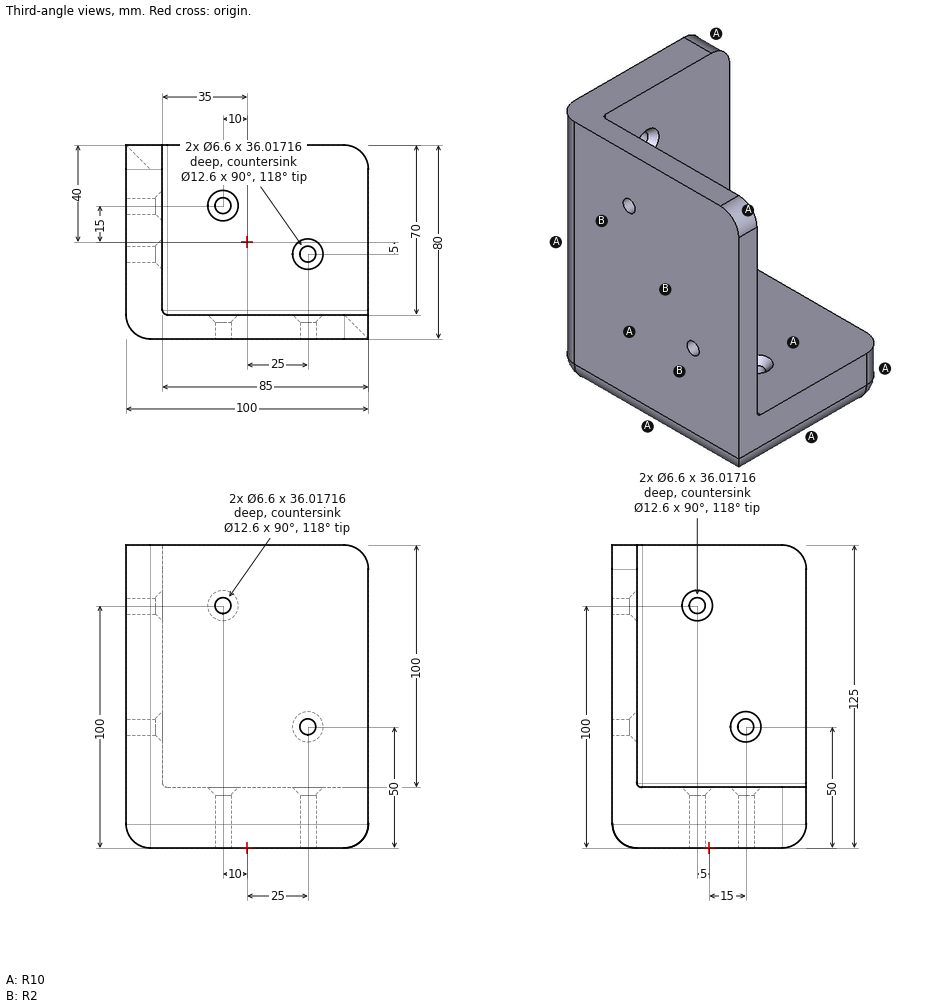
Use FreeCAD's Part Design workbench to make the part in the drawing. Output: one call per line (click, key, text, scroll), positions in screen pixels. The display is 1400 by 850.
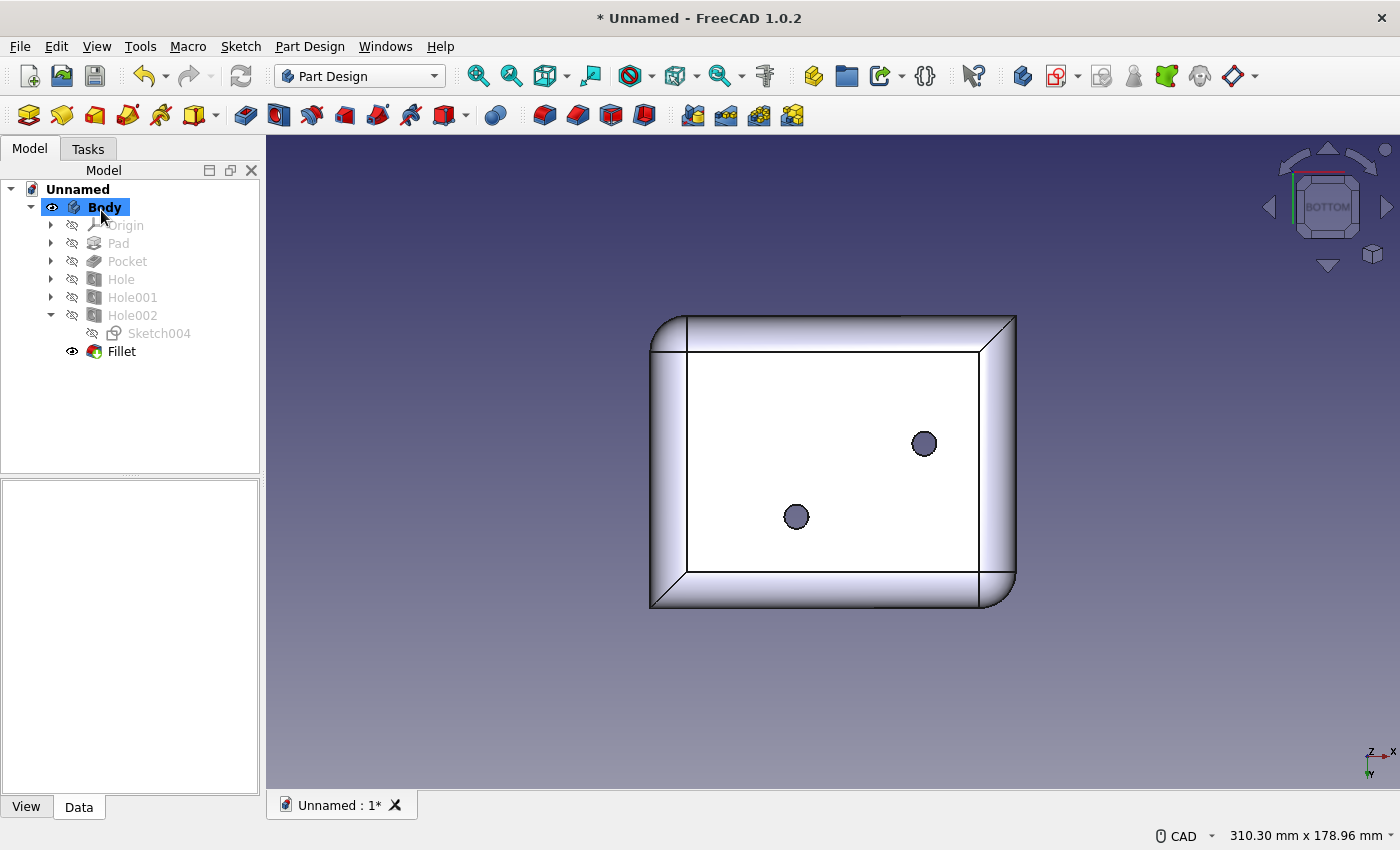
key(0)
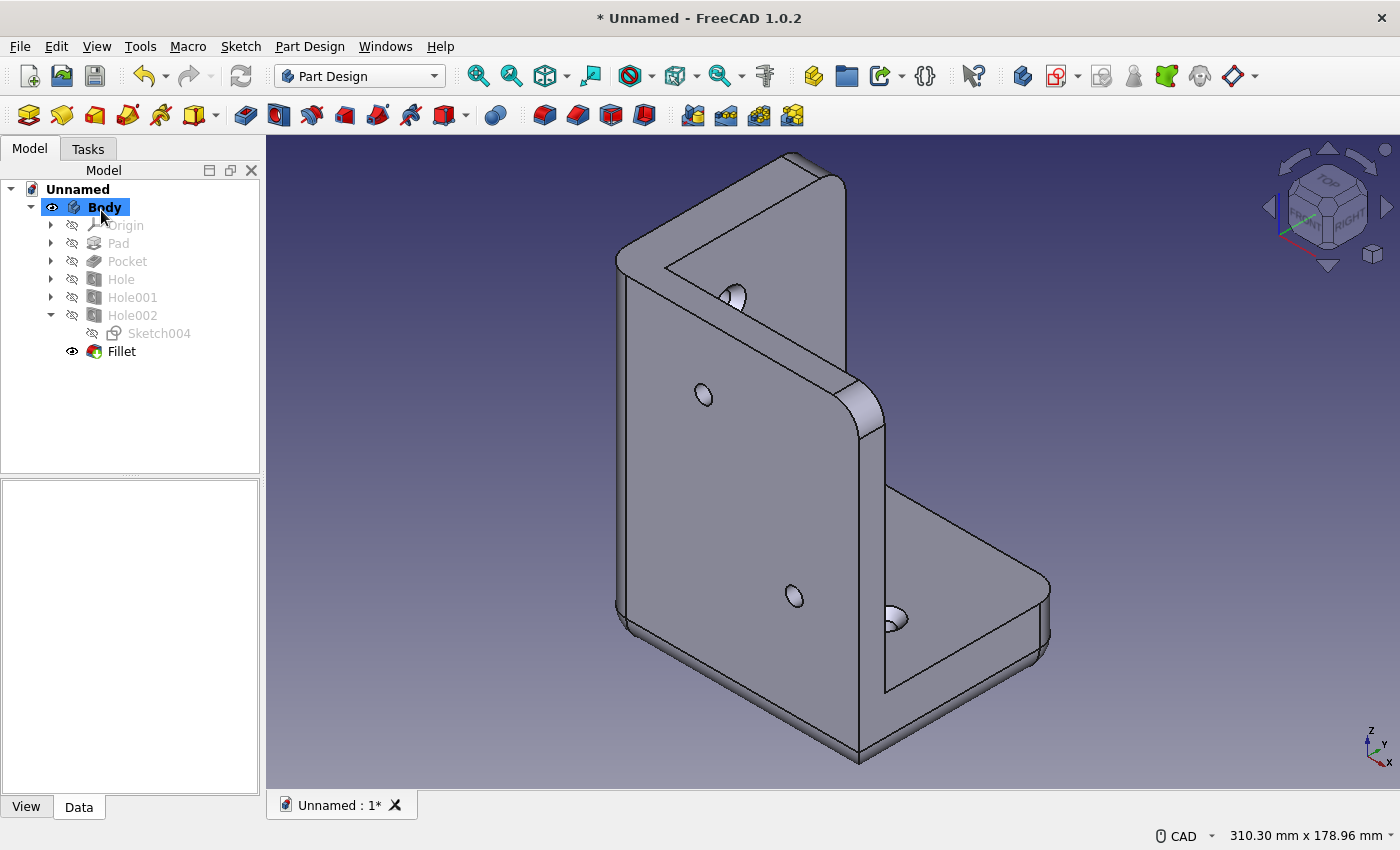
key(2)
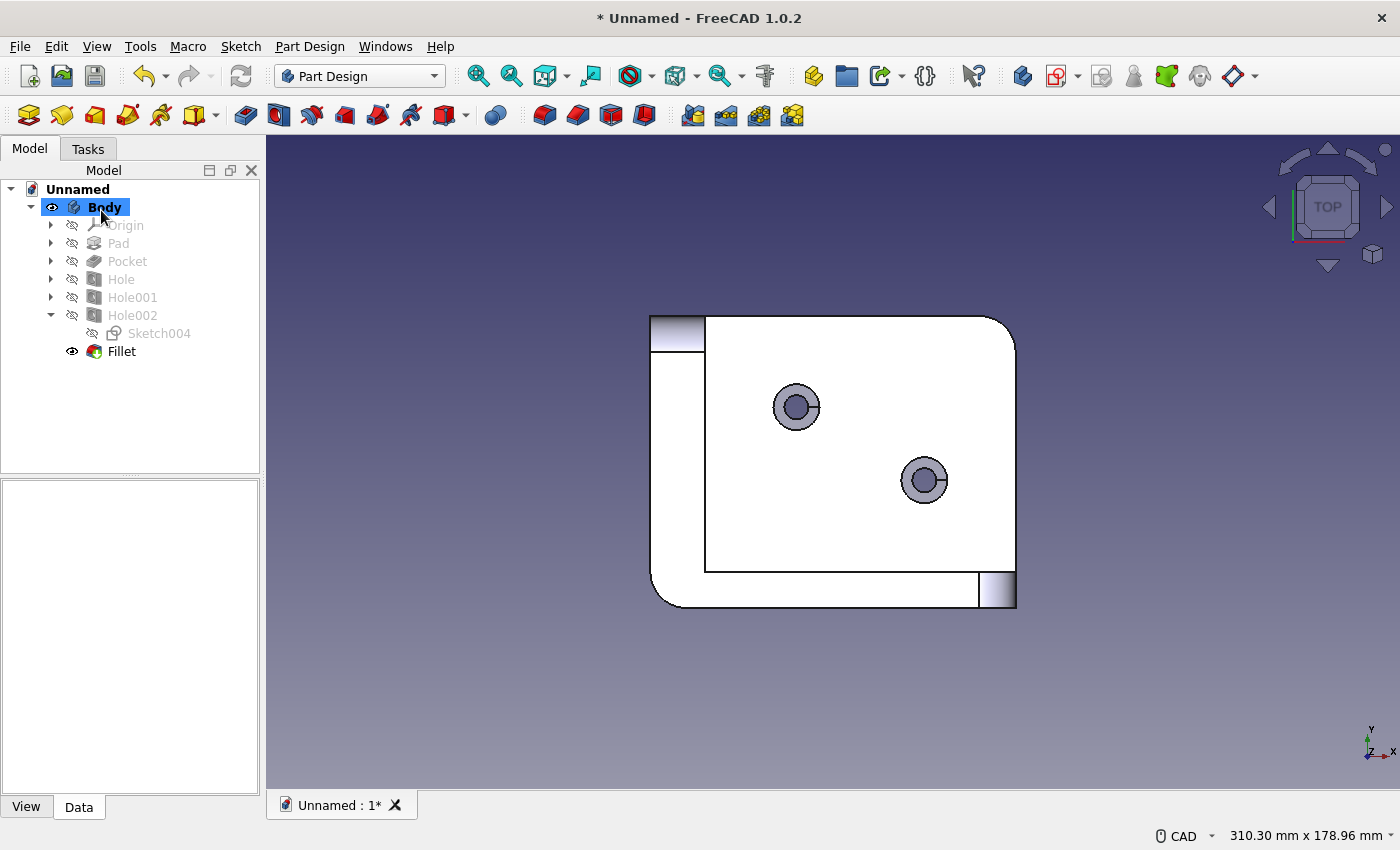
click(479, 76)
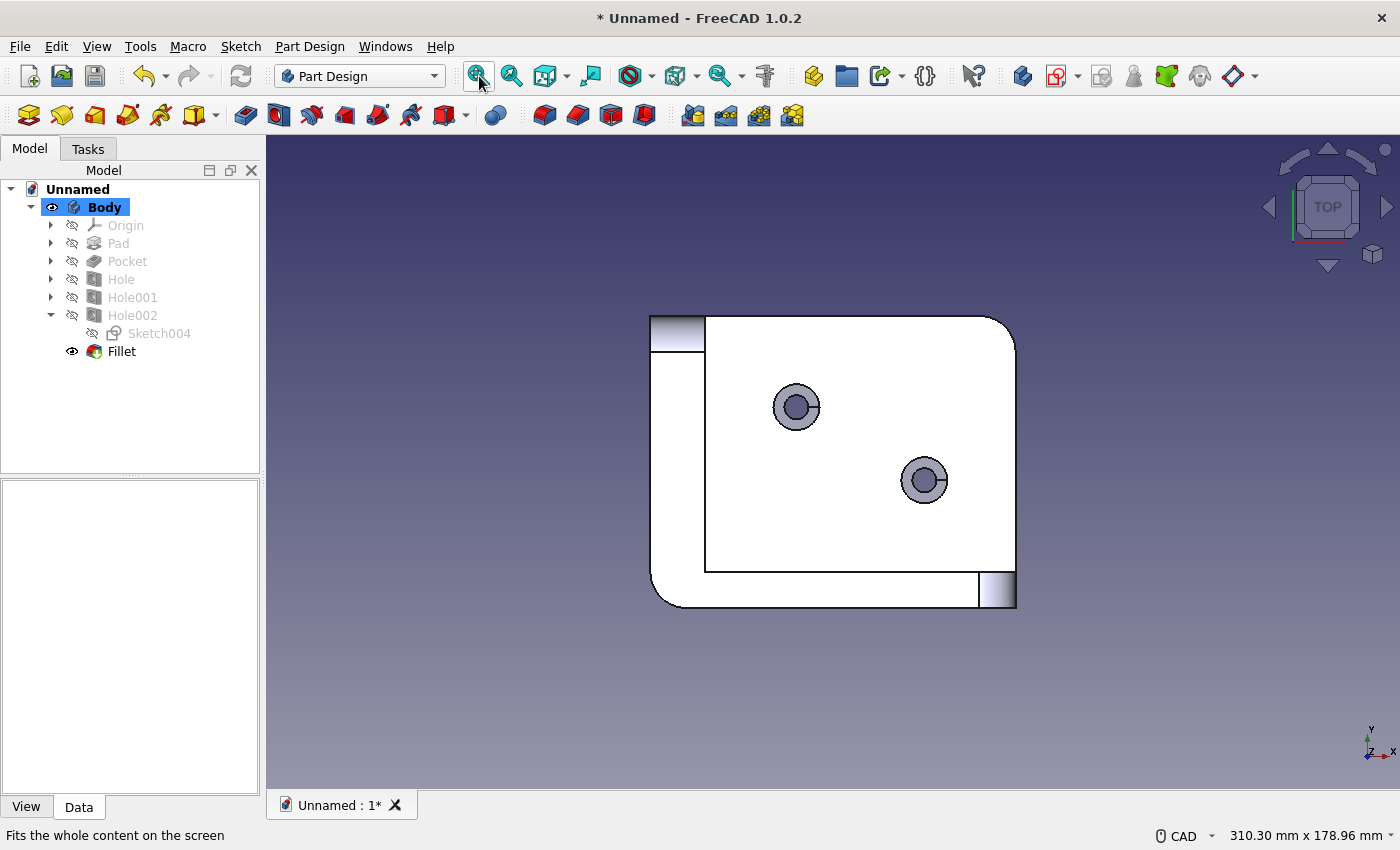
key(1)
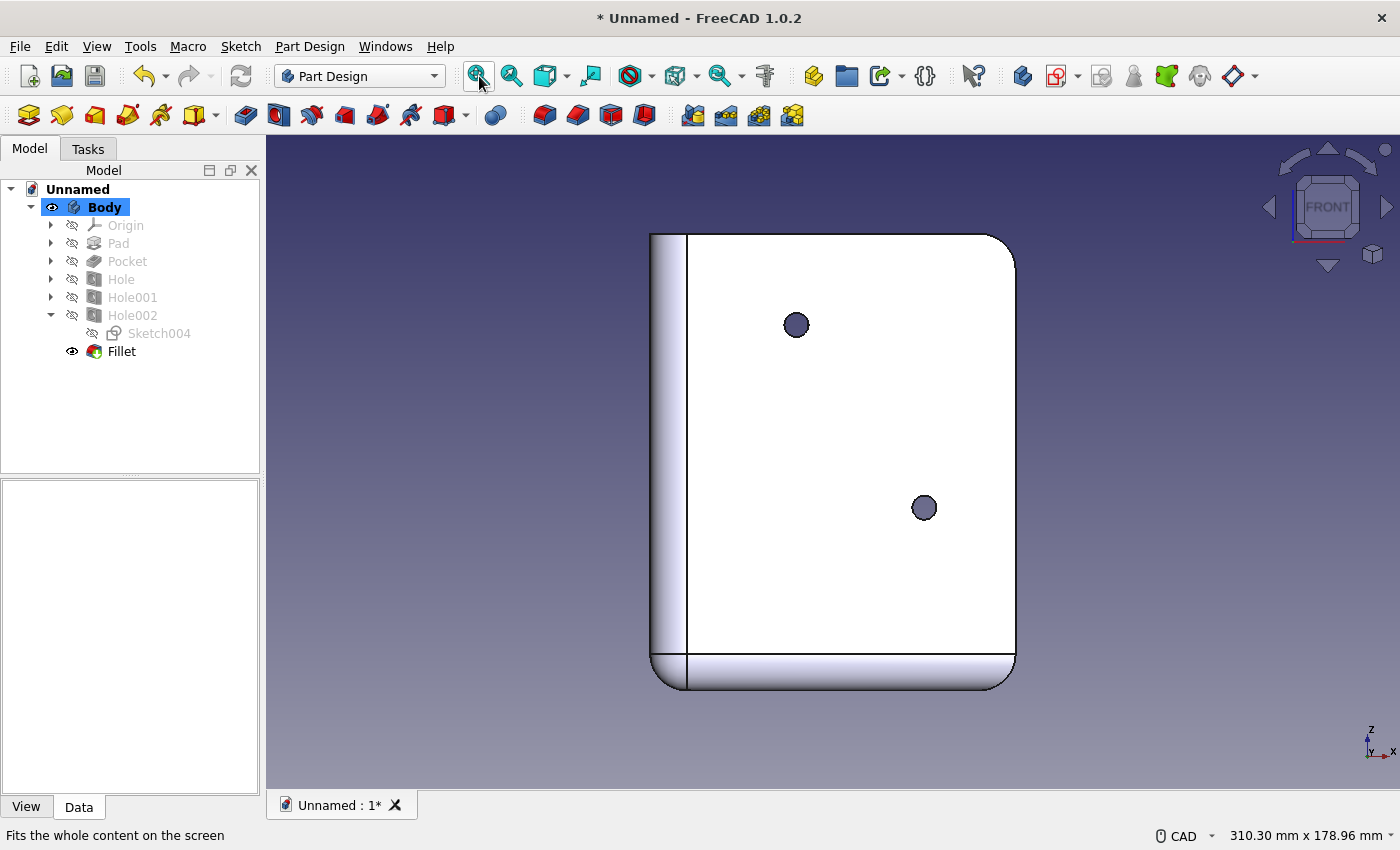
key(3)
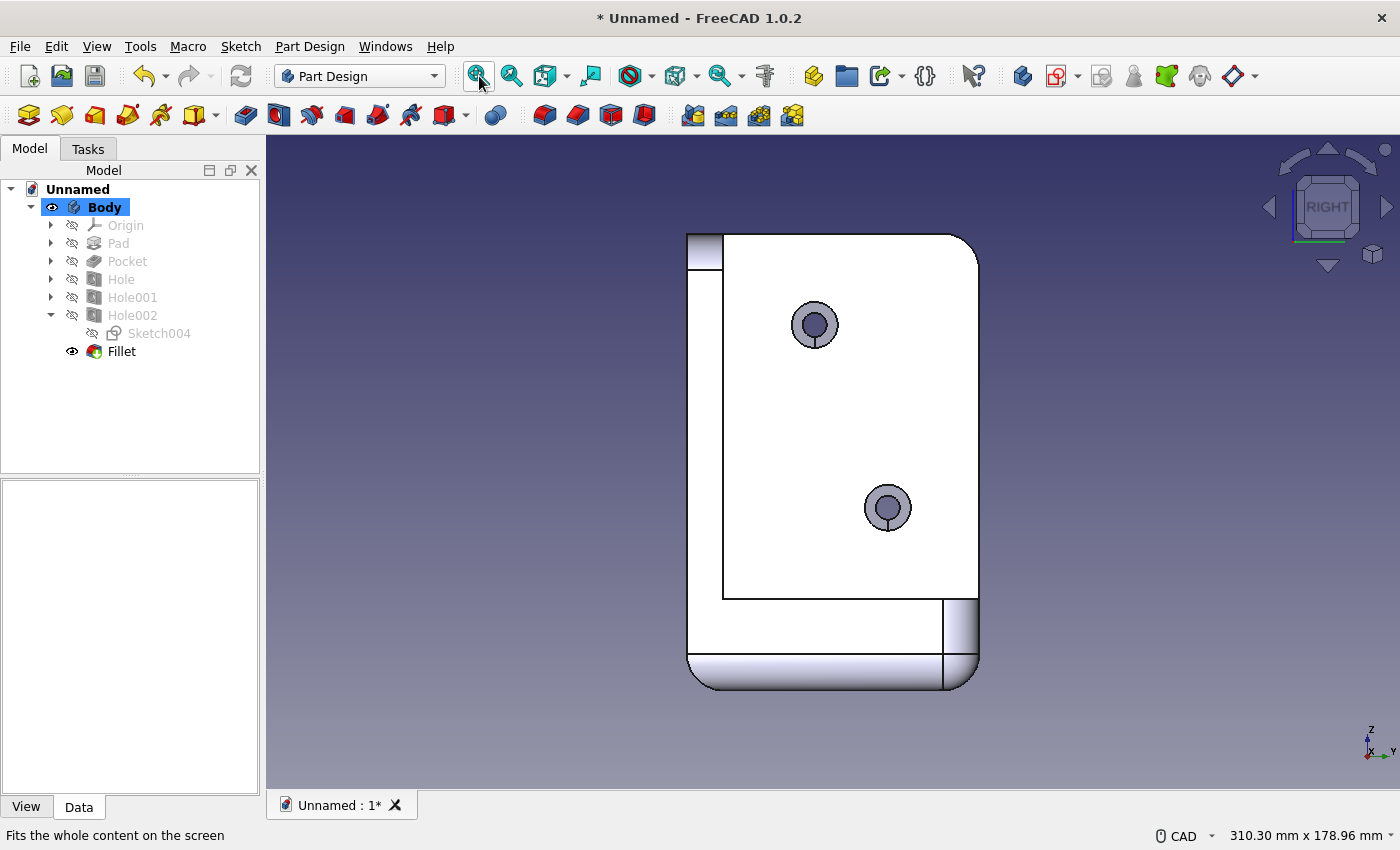
key(5)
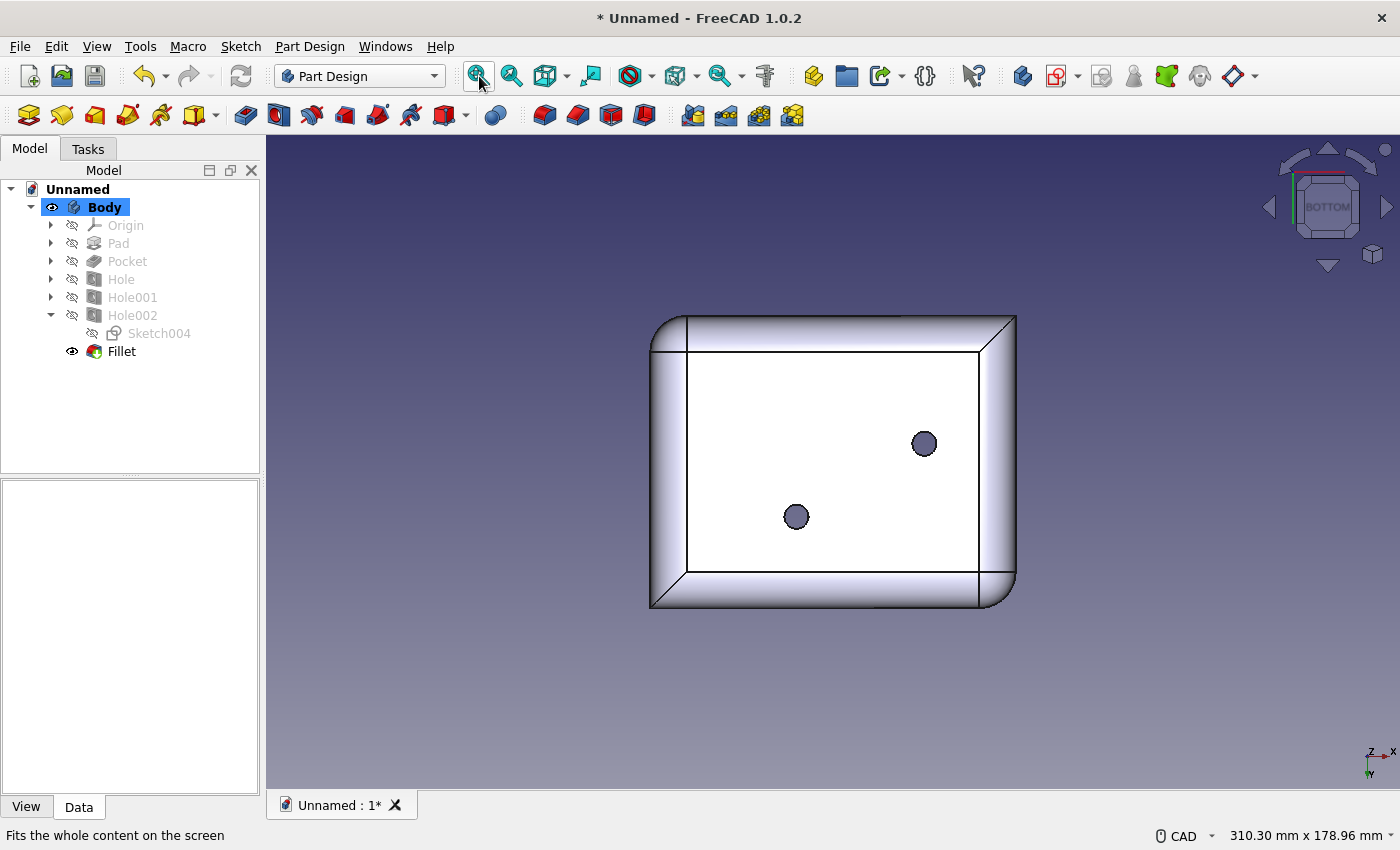
click(479, 76)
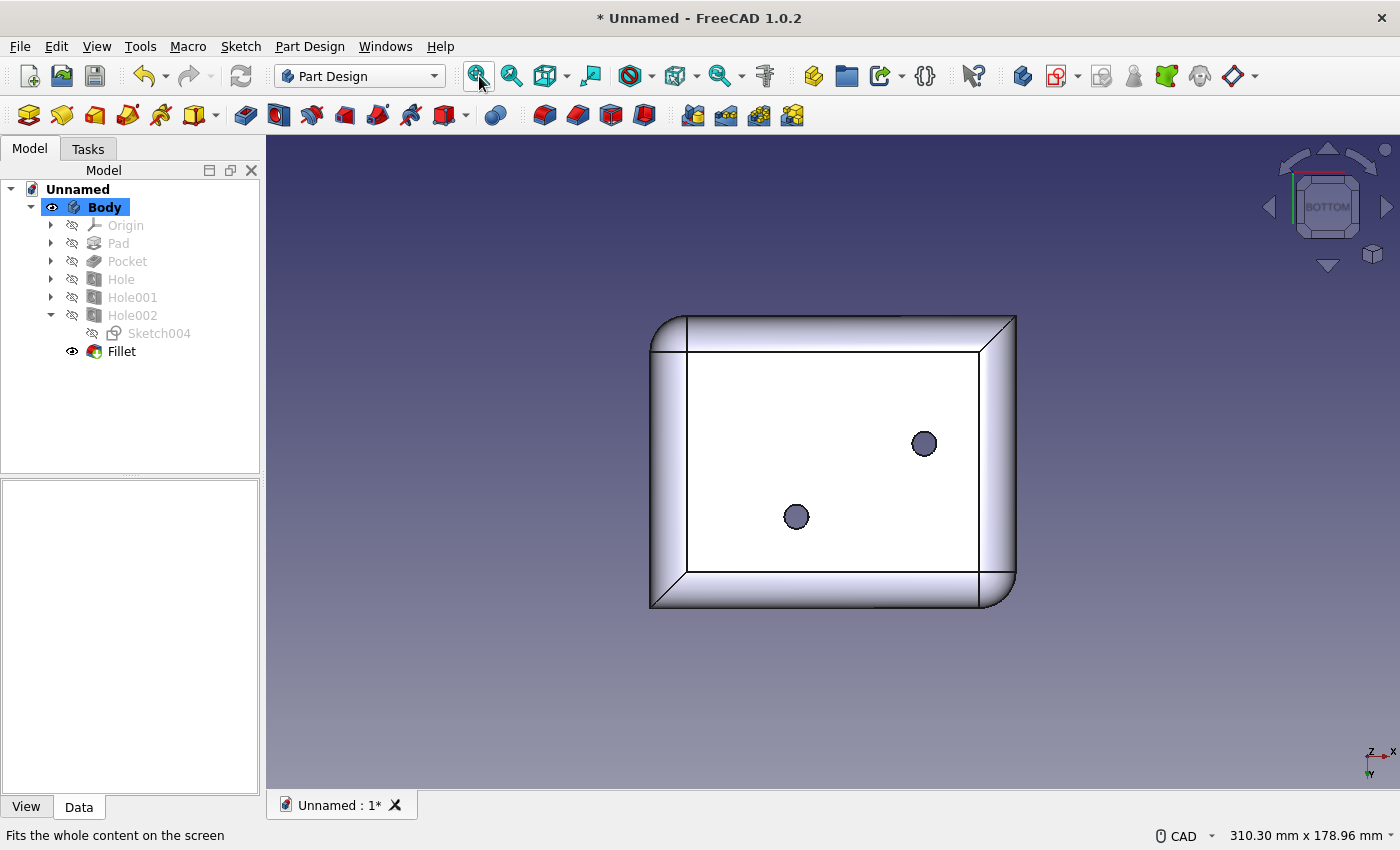
key(4)